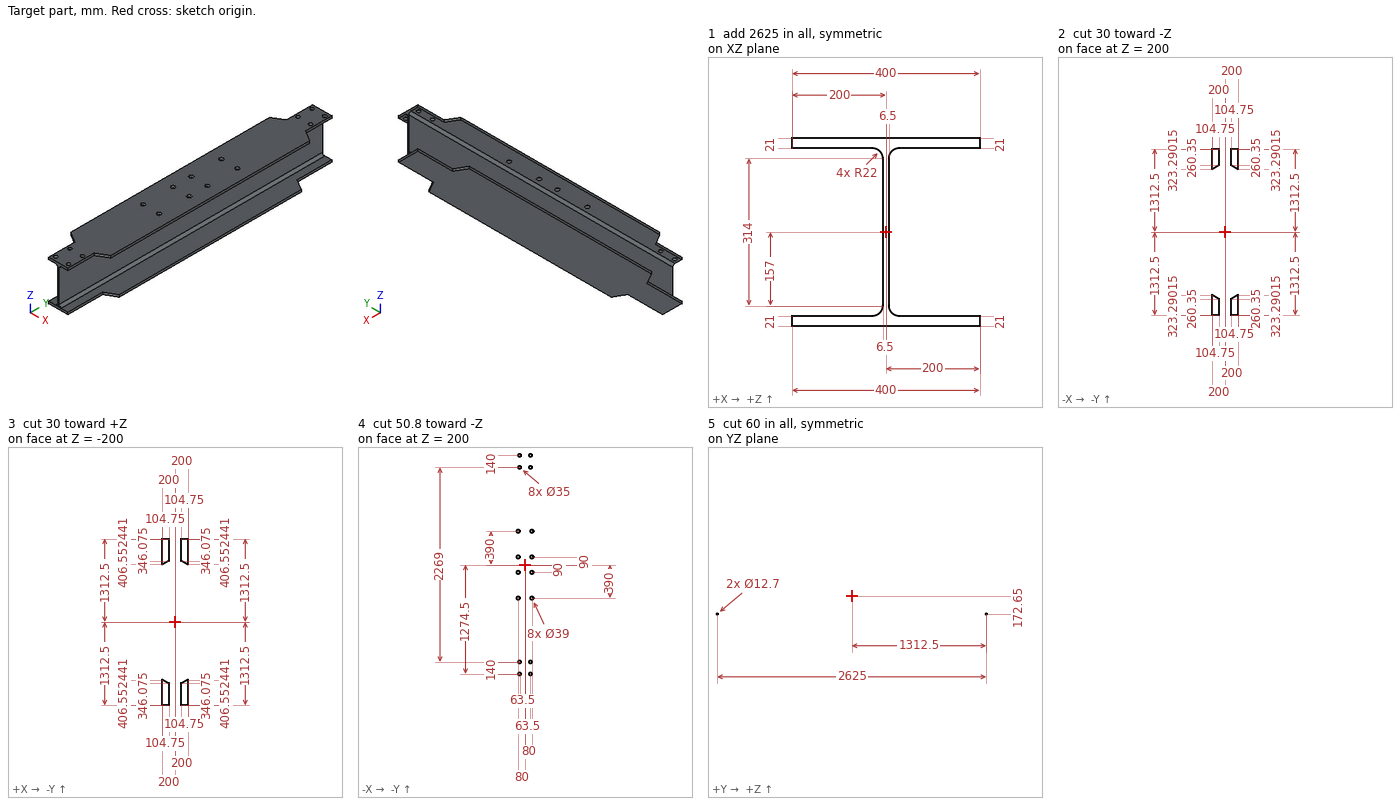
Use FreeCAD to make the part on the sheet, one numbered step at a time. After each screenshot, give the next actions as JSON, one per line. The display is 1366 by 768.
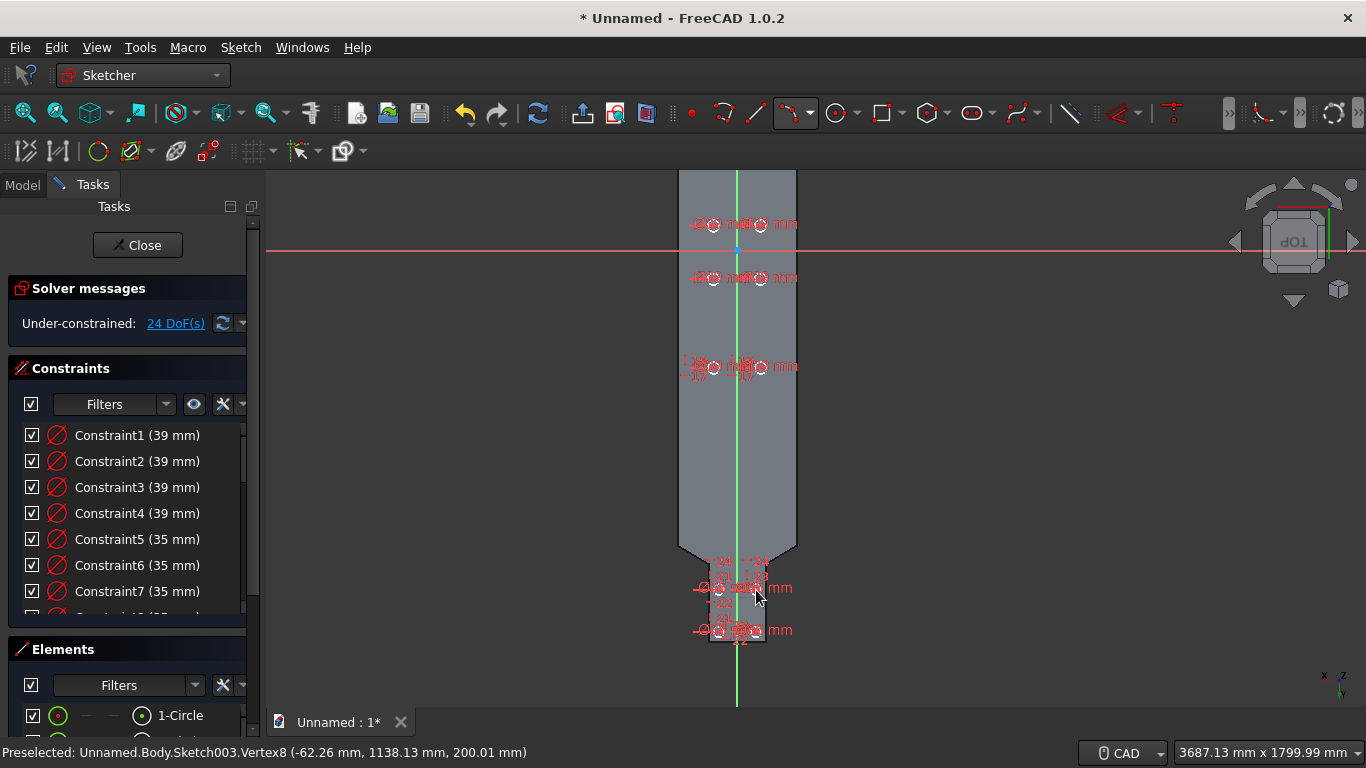
{"action": "left_click", "coordinate": [719, 590]}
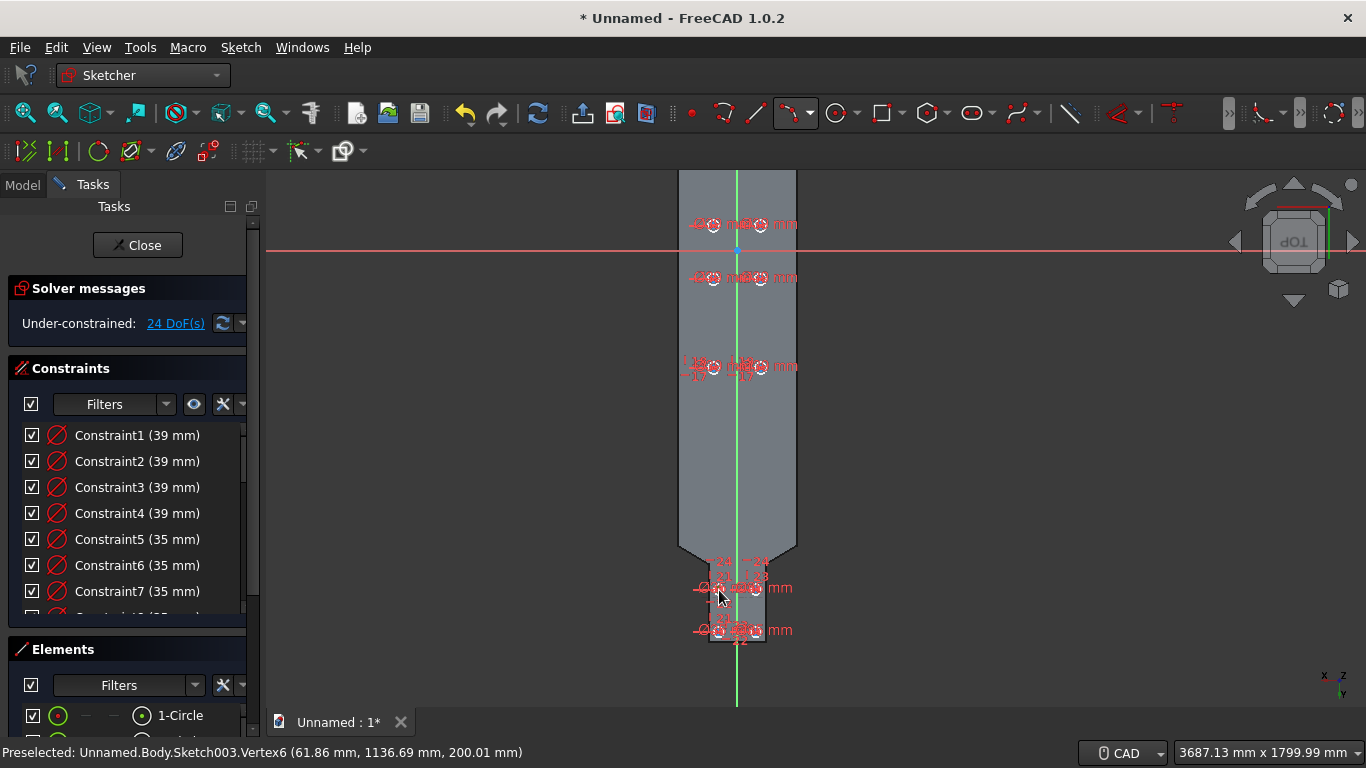
{"action": "scroll", "coordinate": [756, 592], "scroll_direction": "down", "scroll_amount": 4}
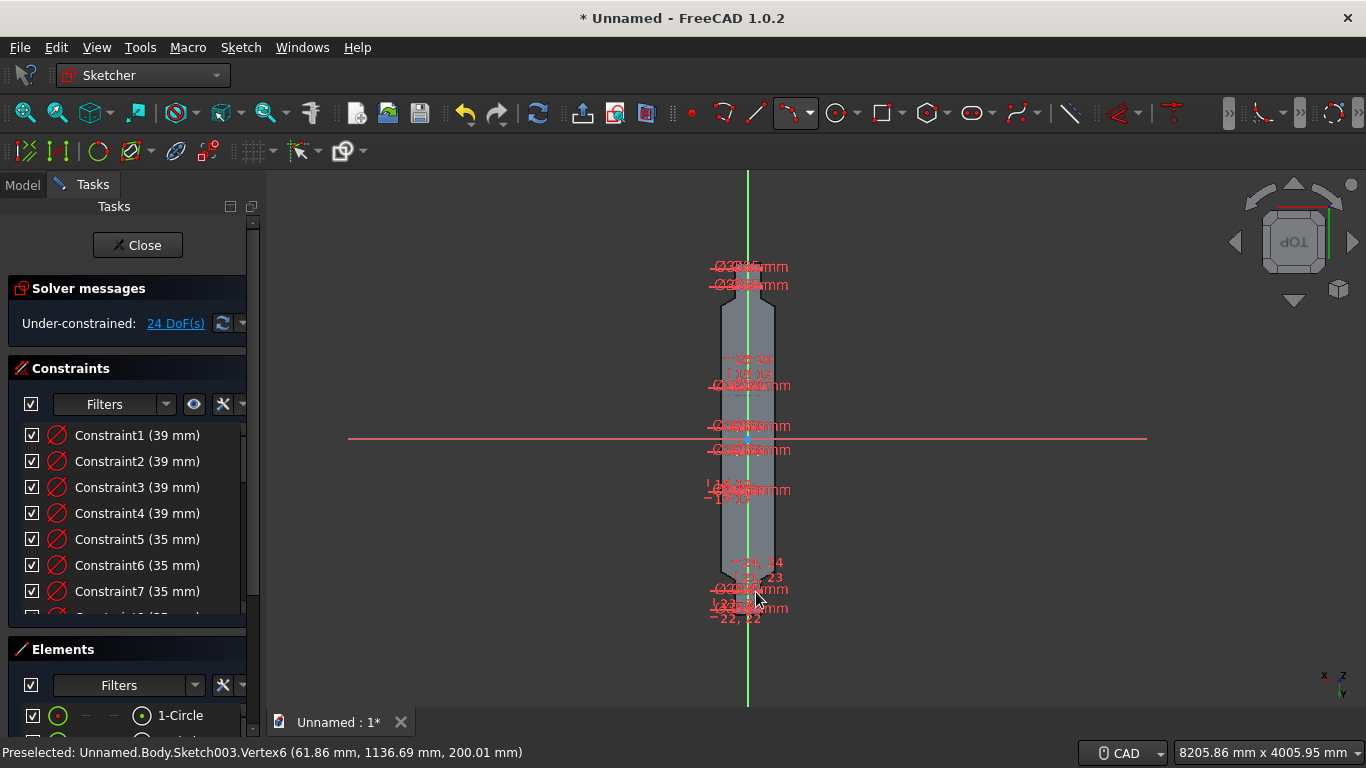
{"action": "left_click", "coordinate": [739, 287]}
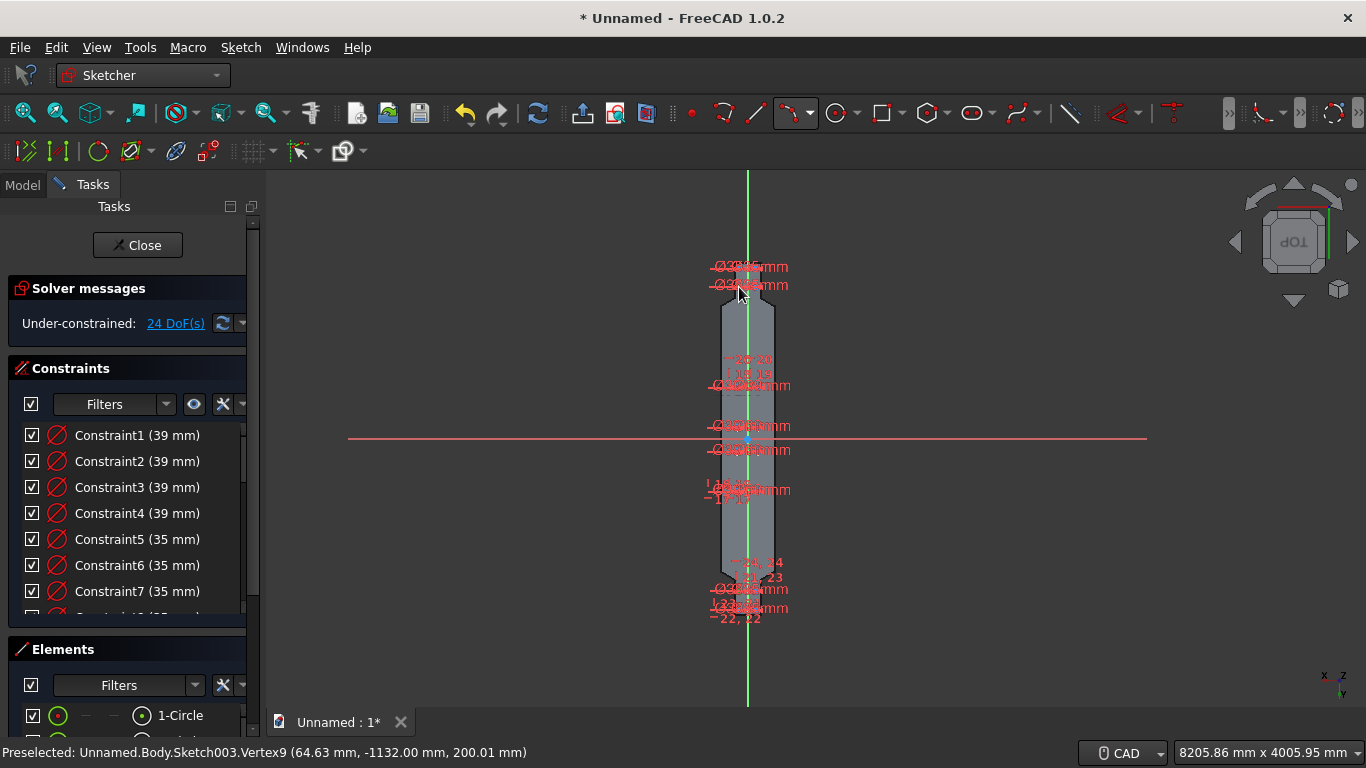
{"action": "key", "text": "v"}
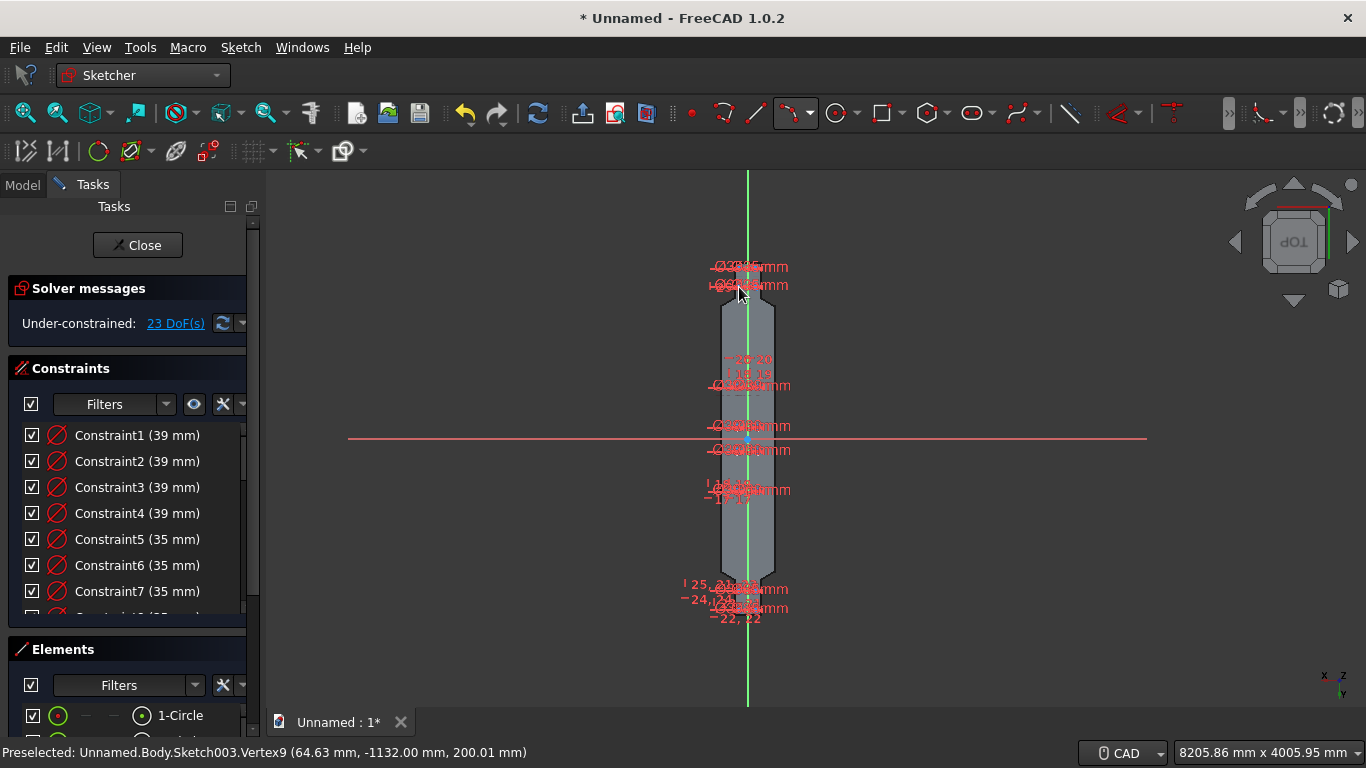
{"action": "left_click", "coordinate": [756, 591]}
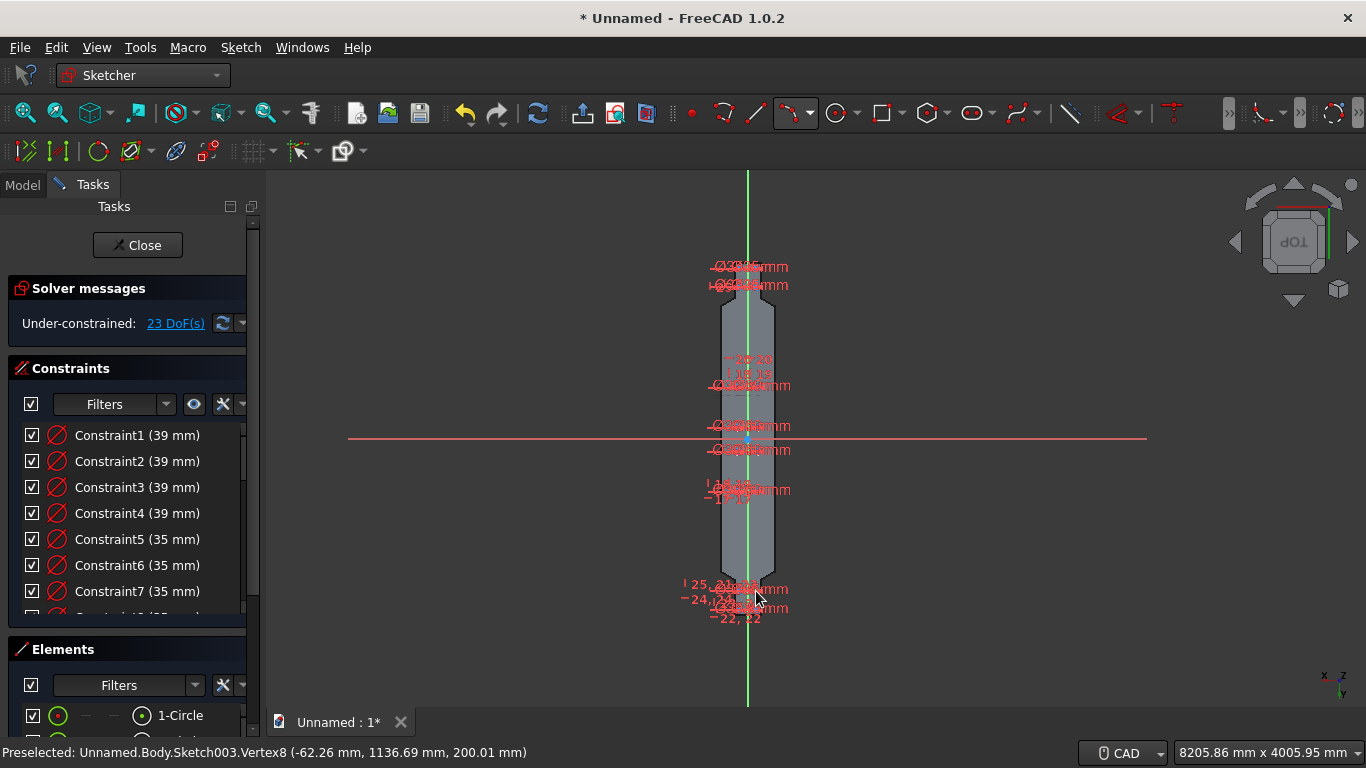
{"action": "left_click", "coordinate": [756, 287]}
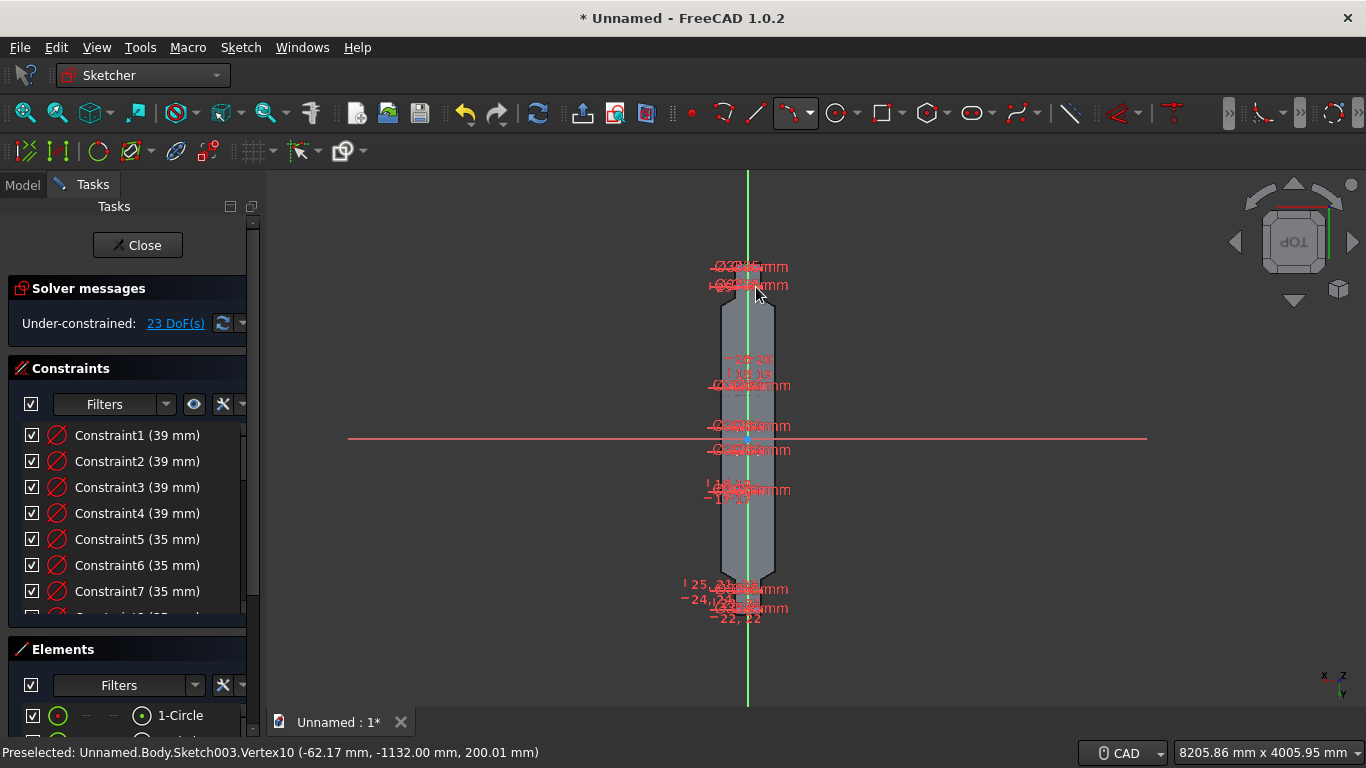
{"action": "key", "text": "v"}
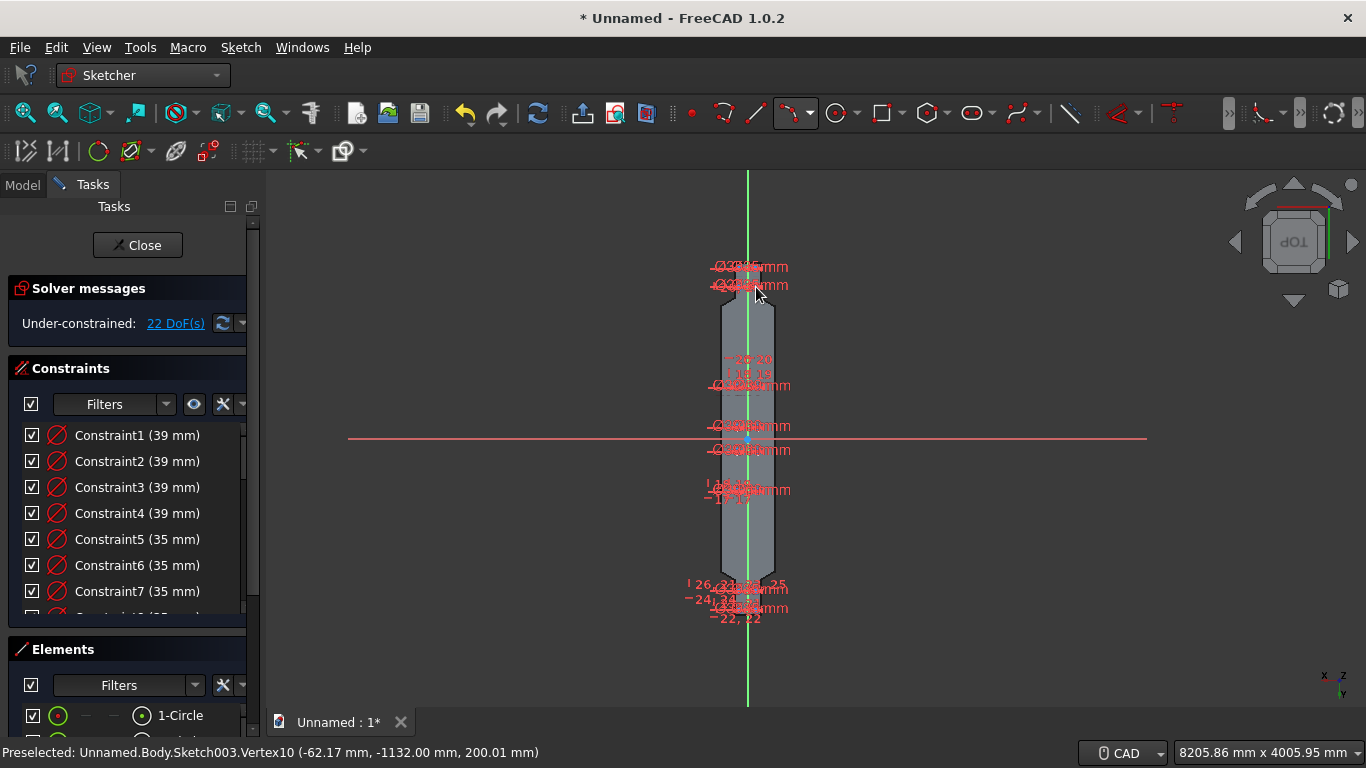
{"action": "scroll", "coordinate": [739, 287], "scroll_direction": "up", "scroll_amount": 4}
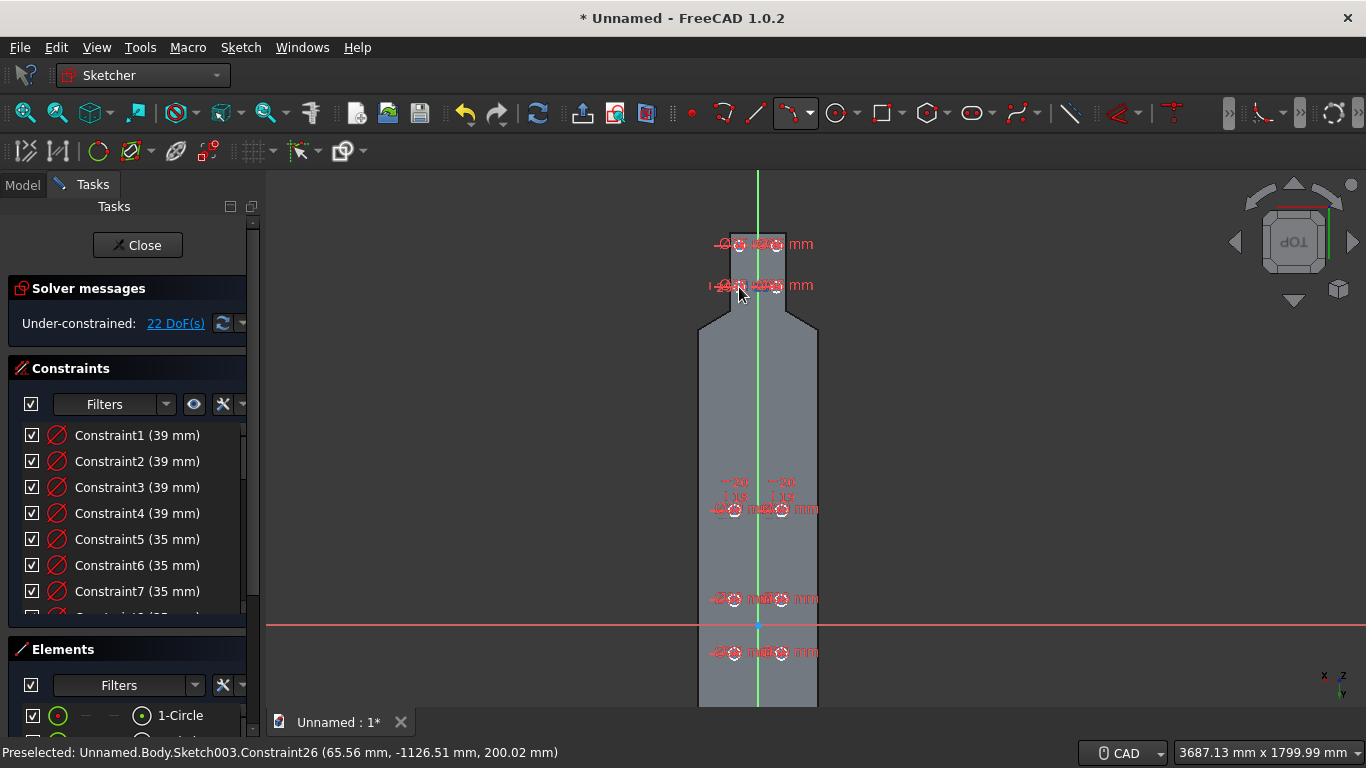
{"action": "left_click", "coordinate": [740, 287]}